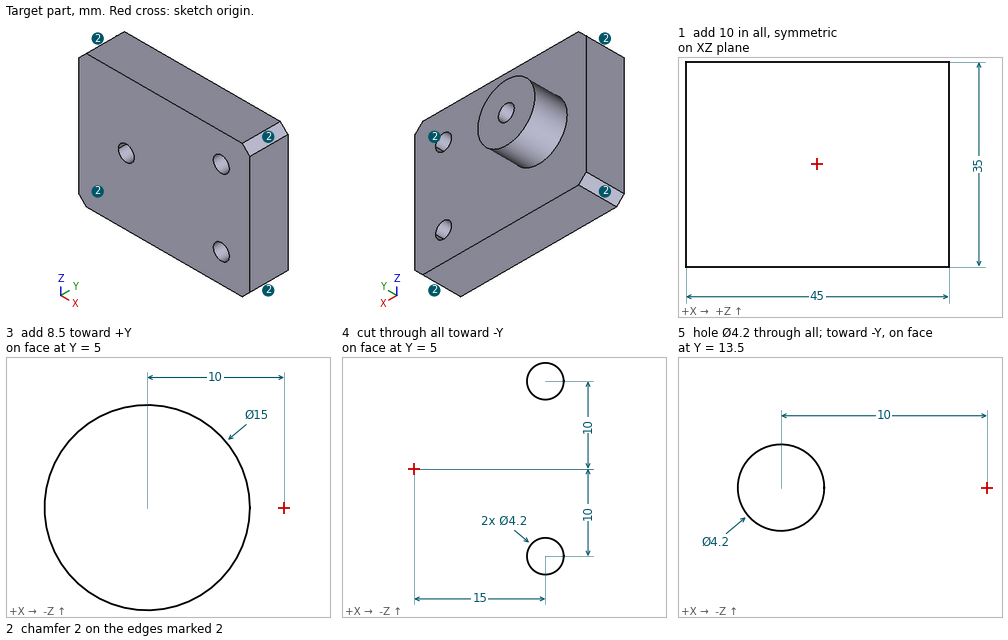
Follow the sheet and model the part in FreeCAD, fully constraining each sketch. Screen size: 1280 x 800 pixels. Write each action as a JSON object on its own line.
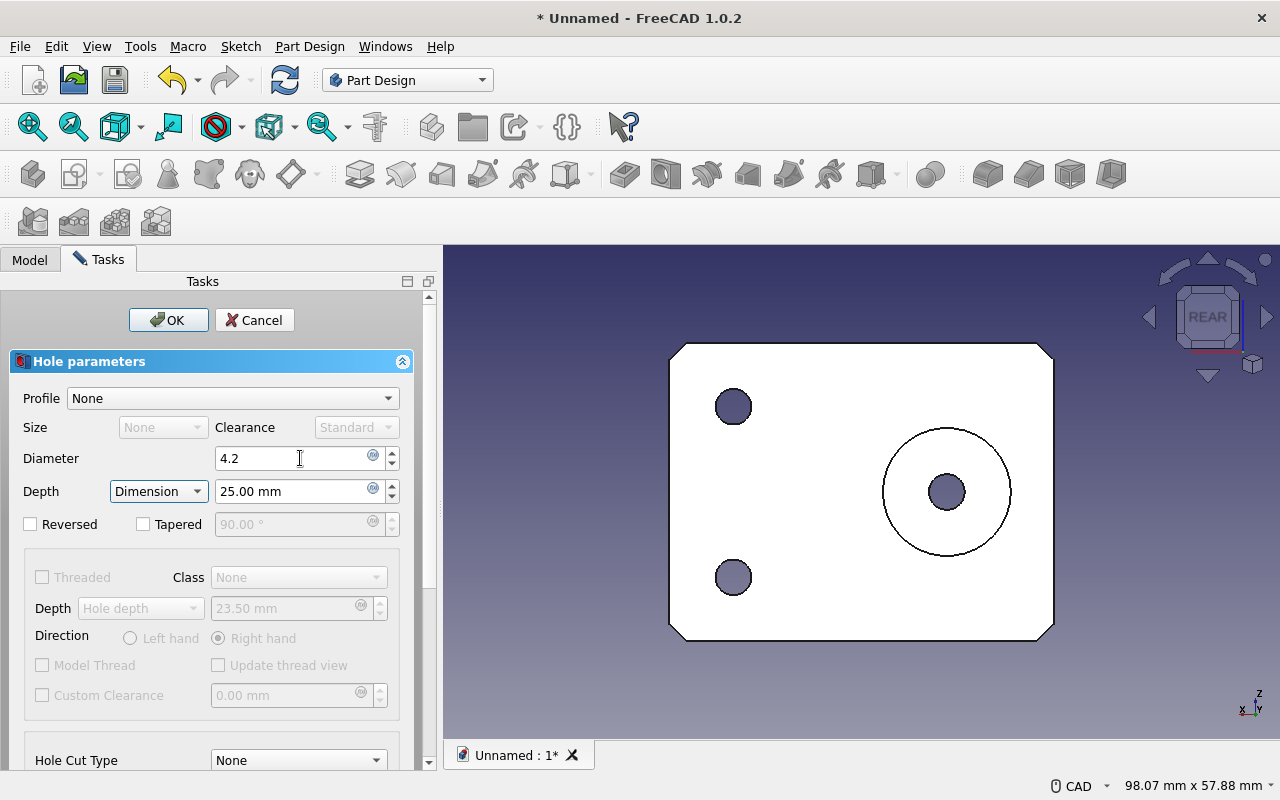
{"action": "left_click", "coordinate": [160, 492]}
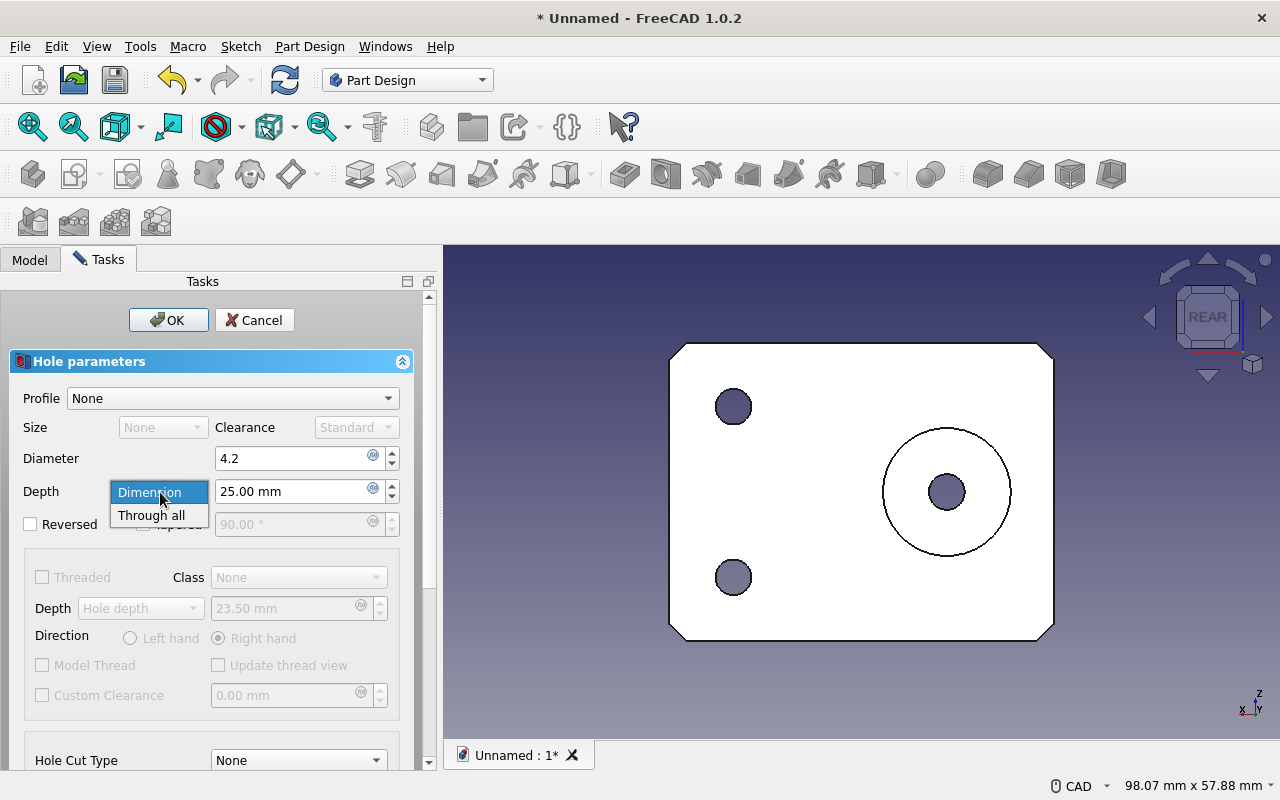
{"action": "left_click", "coordinate": [158, 516]}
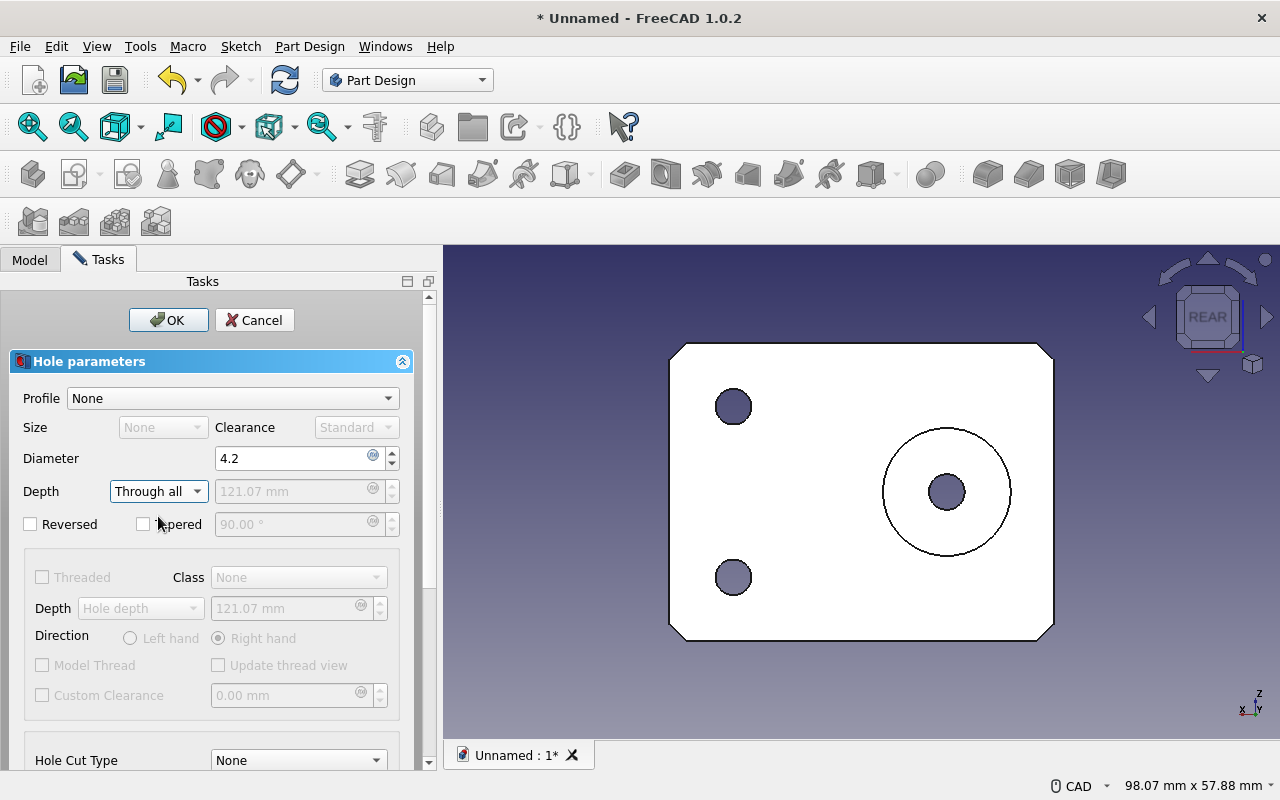
{"action": "left_click", "coordinate": [169, 320]}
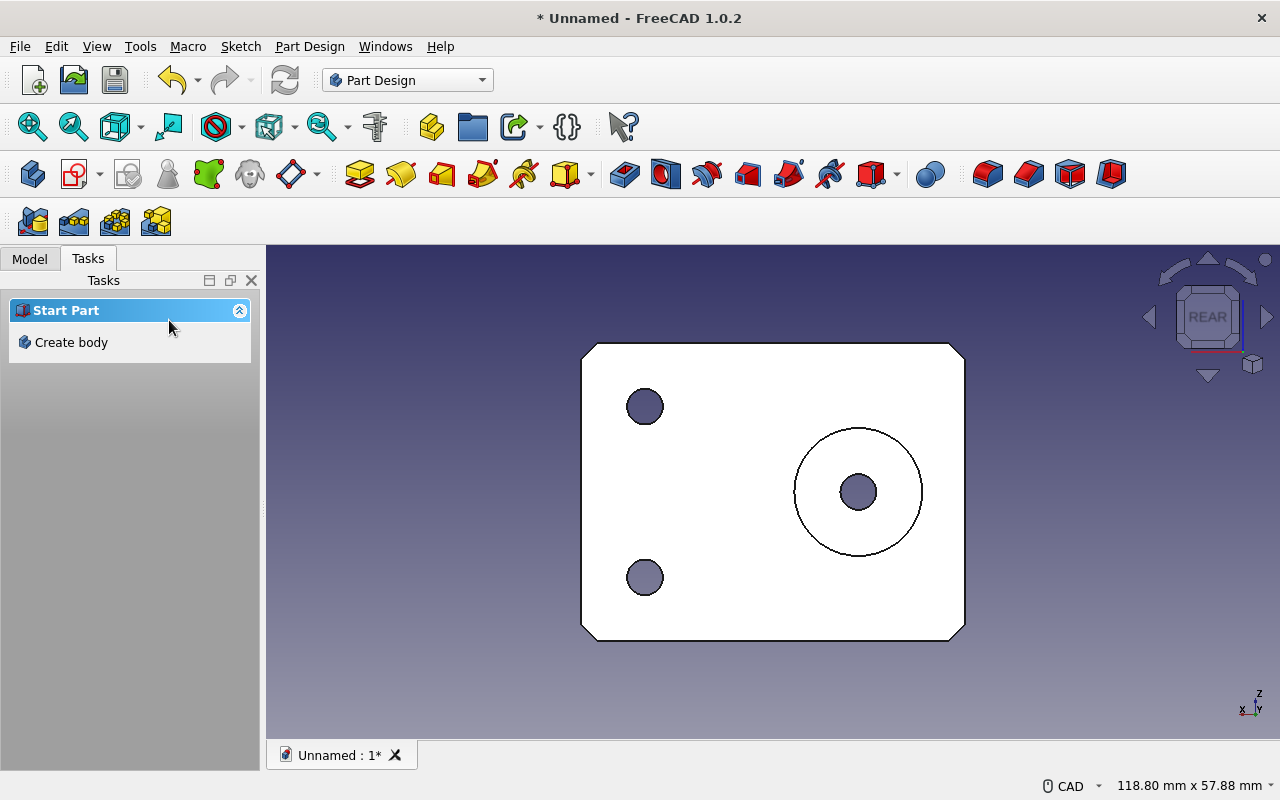
{"action": "key", "text": "0"}